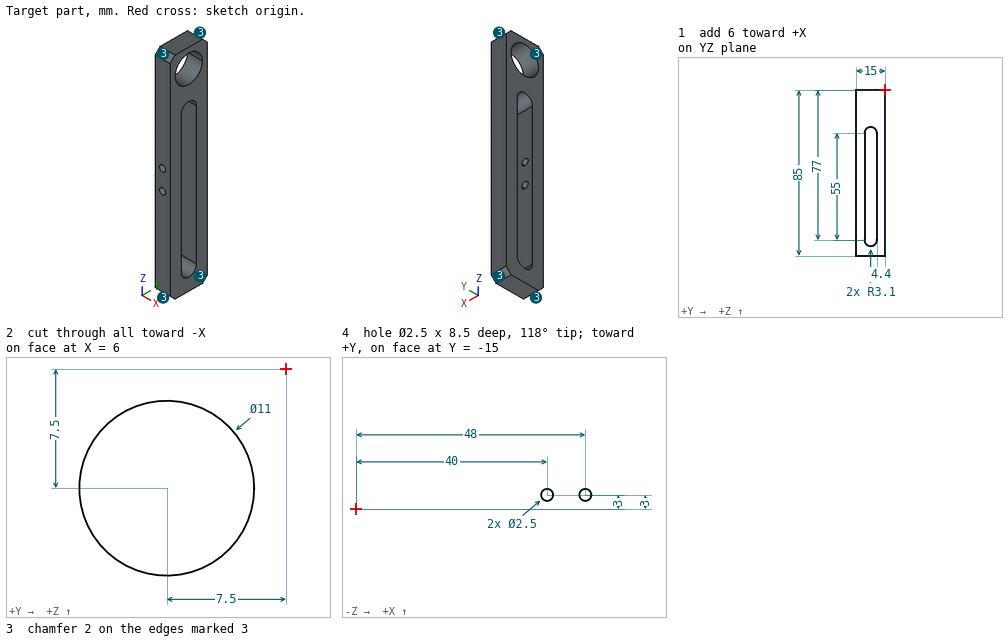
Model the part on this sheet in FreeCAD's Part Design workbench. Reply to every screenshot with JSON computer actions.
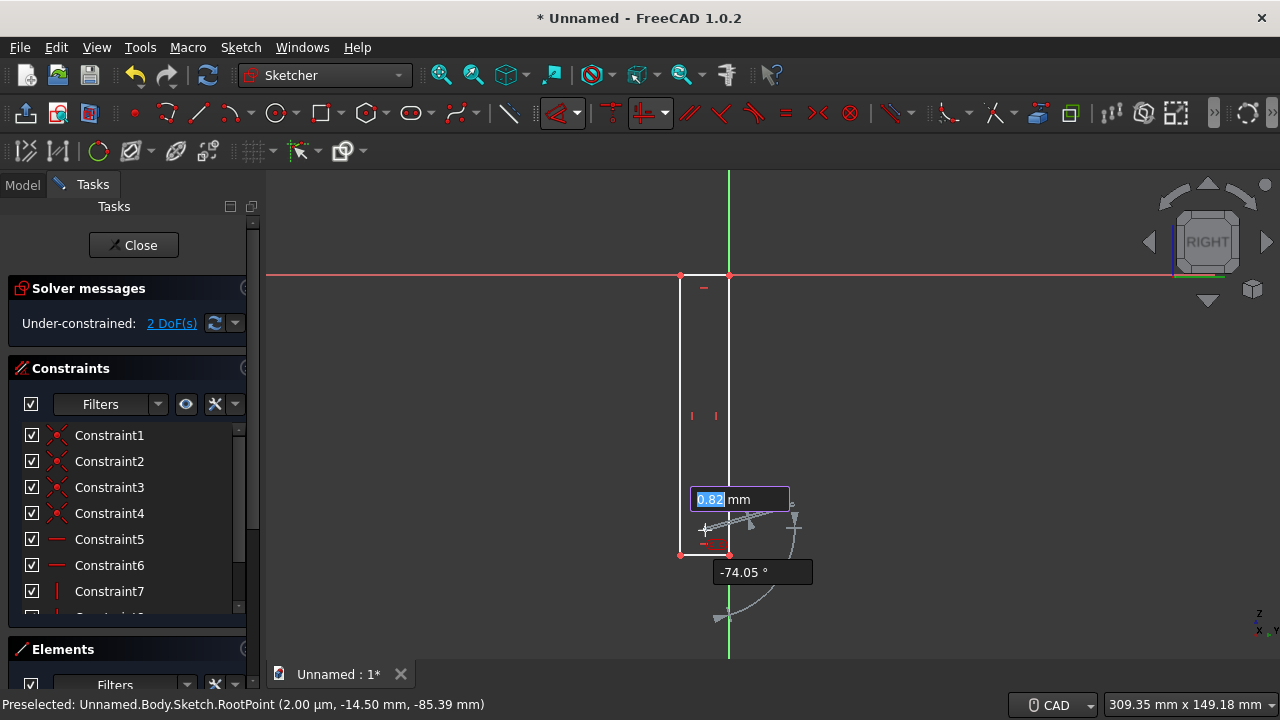
{"action": "left_click", "coordinate": [705, 348]}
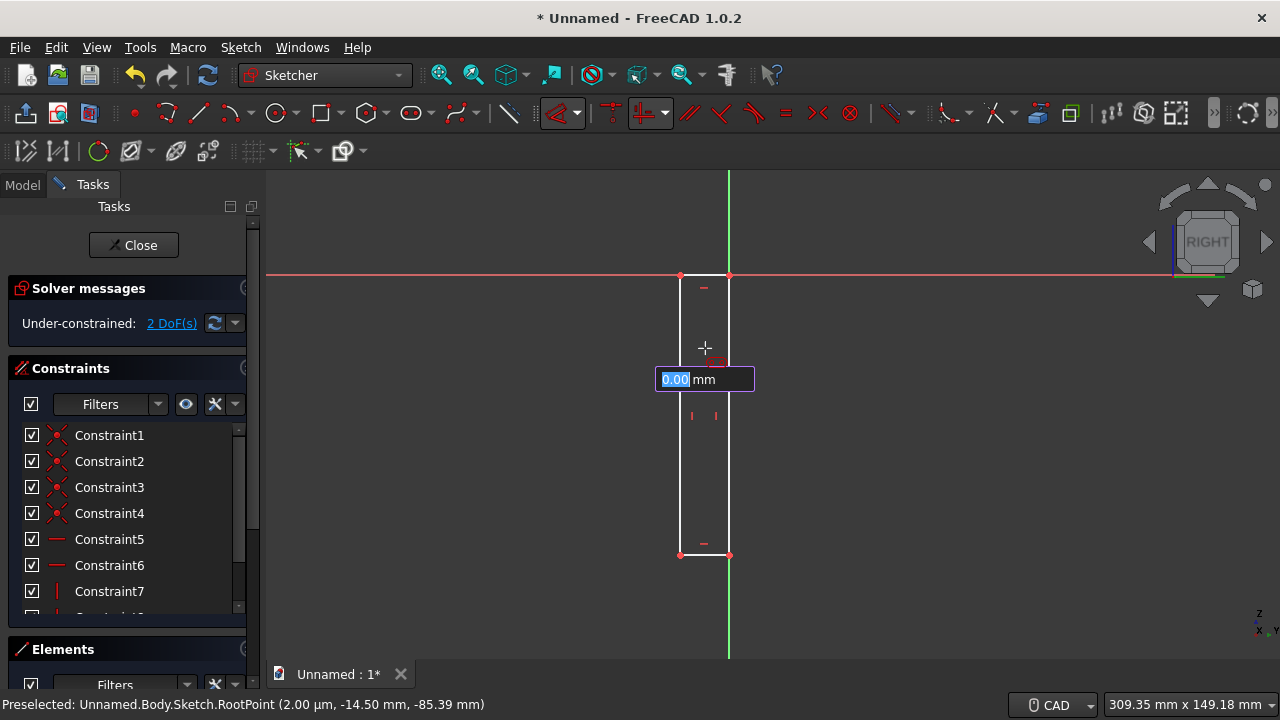
{"action": "scroll", "coordinate": [715, 438], "scroll_direction": "up", "scroll_amount": 3}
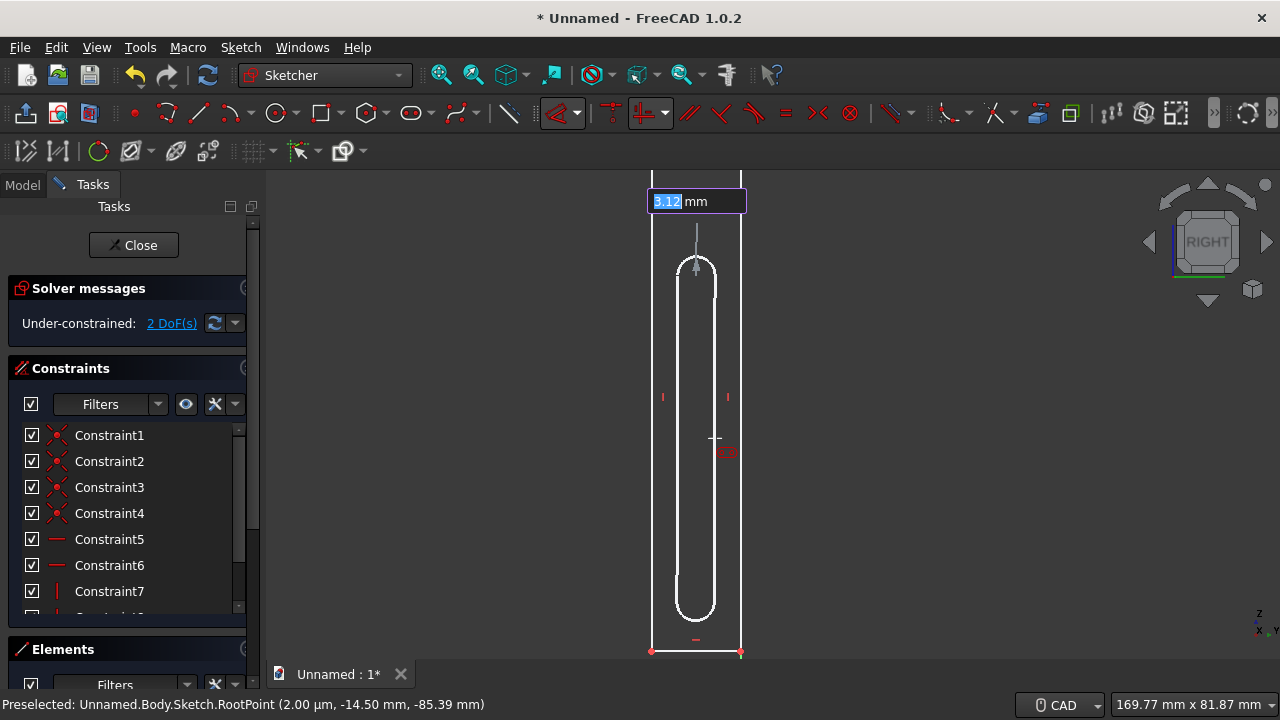
{"action": "left_click", "coordinate": [714, 437]}
{"action": "key", "text": "Escape"}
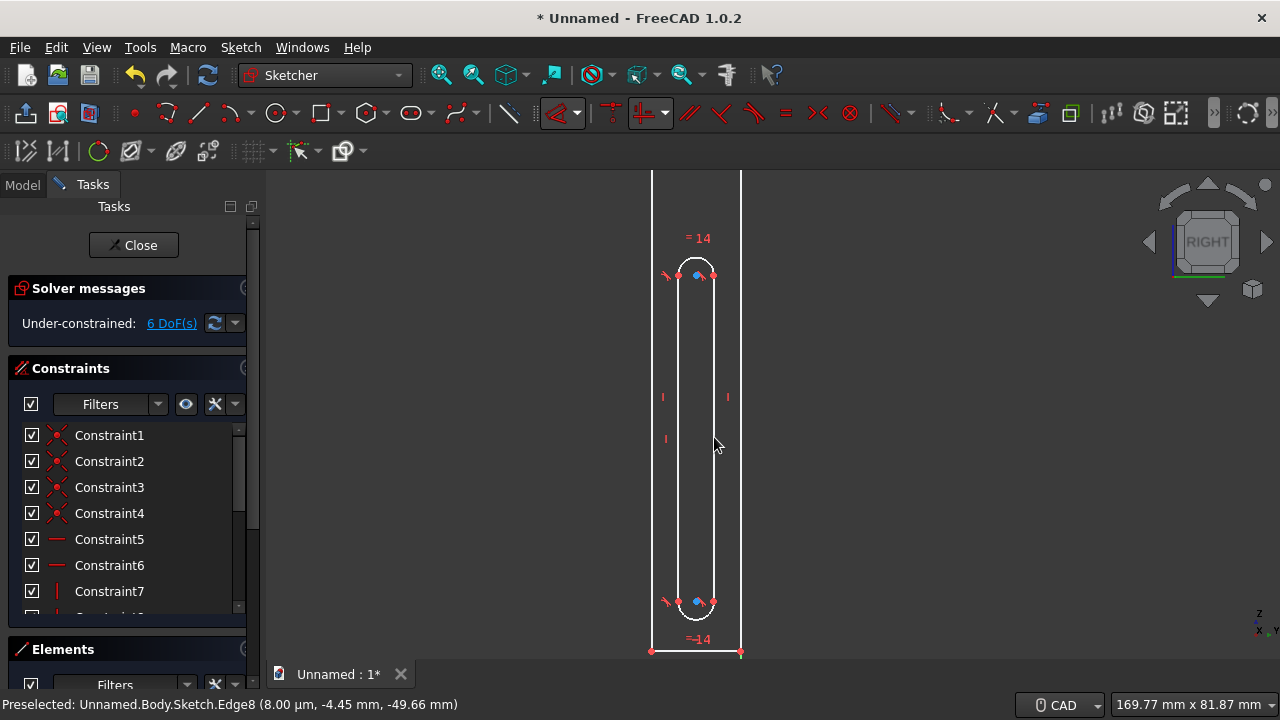
{"action": "key", "text": "d"}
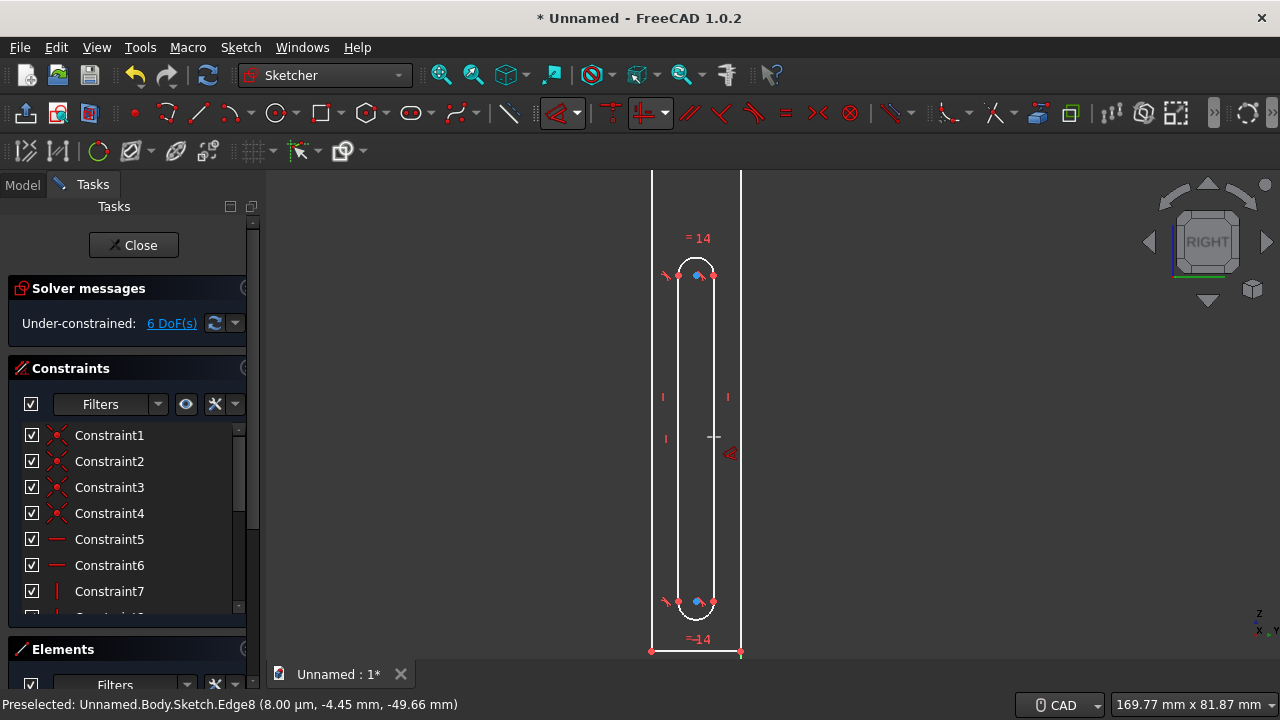
{"action": "scroll", "coordinate": [686, 616], "scroll_direction": "up", "scroll_amount": 4}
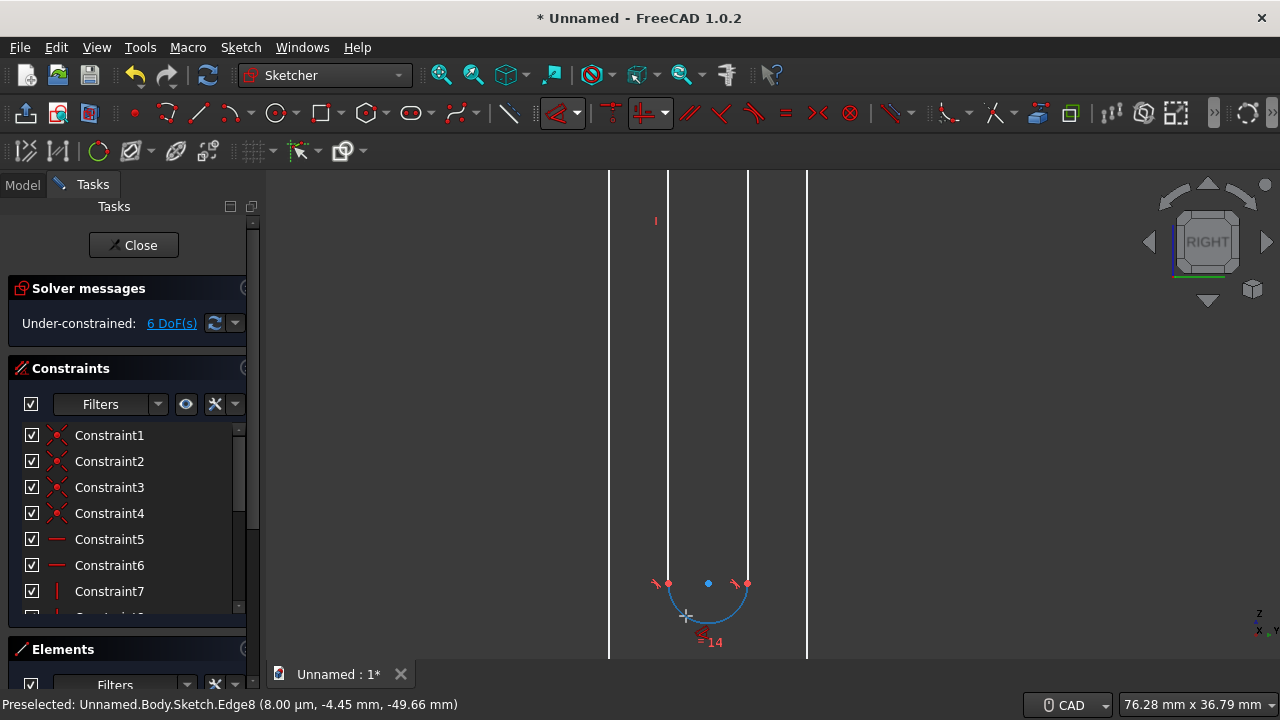
{"action": "left_click", "coordinate": [685, 616]}
{"action": "left_click", "coordinate": [644, 615]}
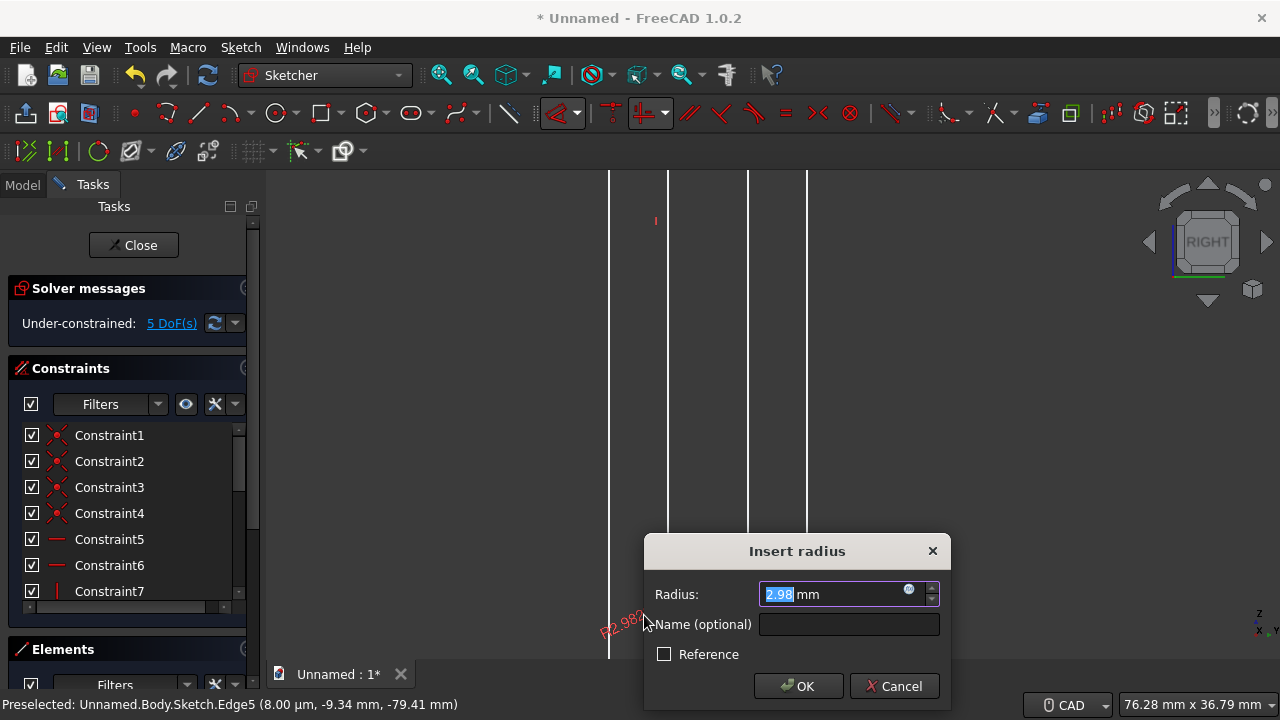
{"action": "type", "text": "3.1"}
{"action": "key", "text": "Return"}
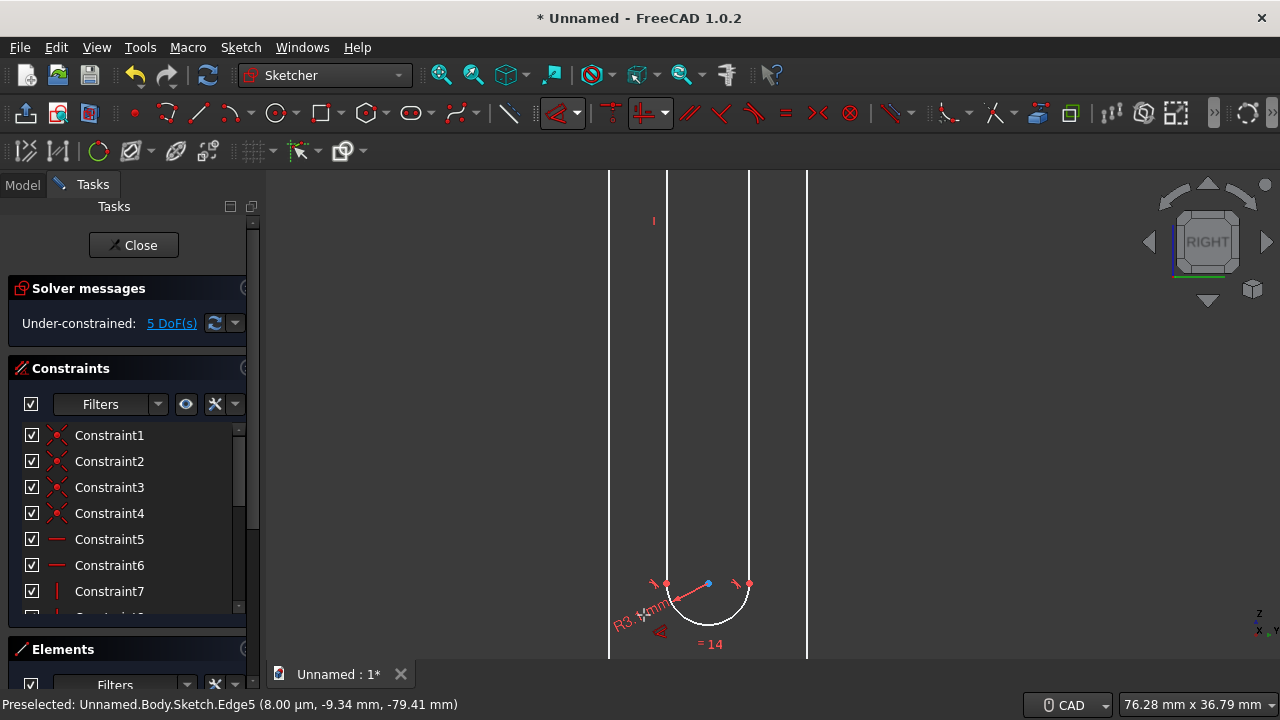
{"action": "scroll", "coordinate": [704, 510], "scroll_direction": "down", "scroll_amount": 7}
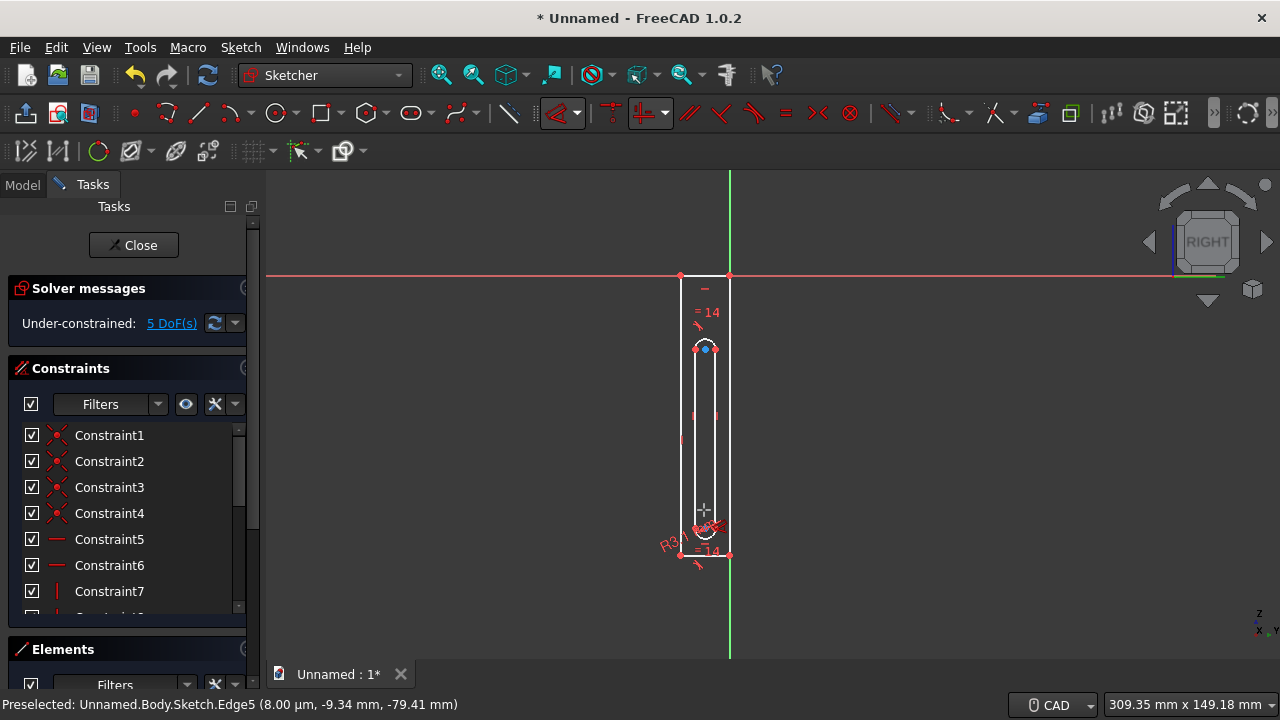
{"action": "left_click", "coordinate": [715, 276]}
{"action": "left_click", "coordinate": [705, 242]}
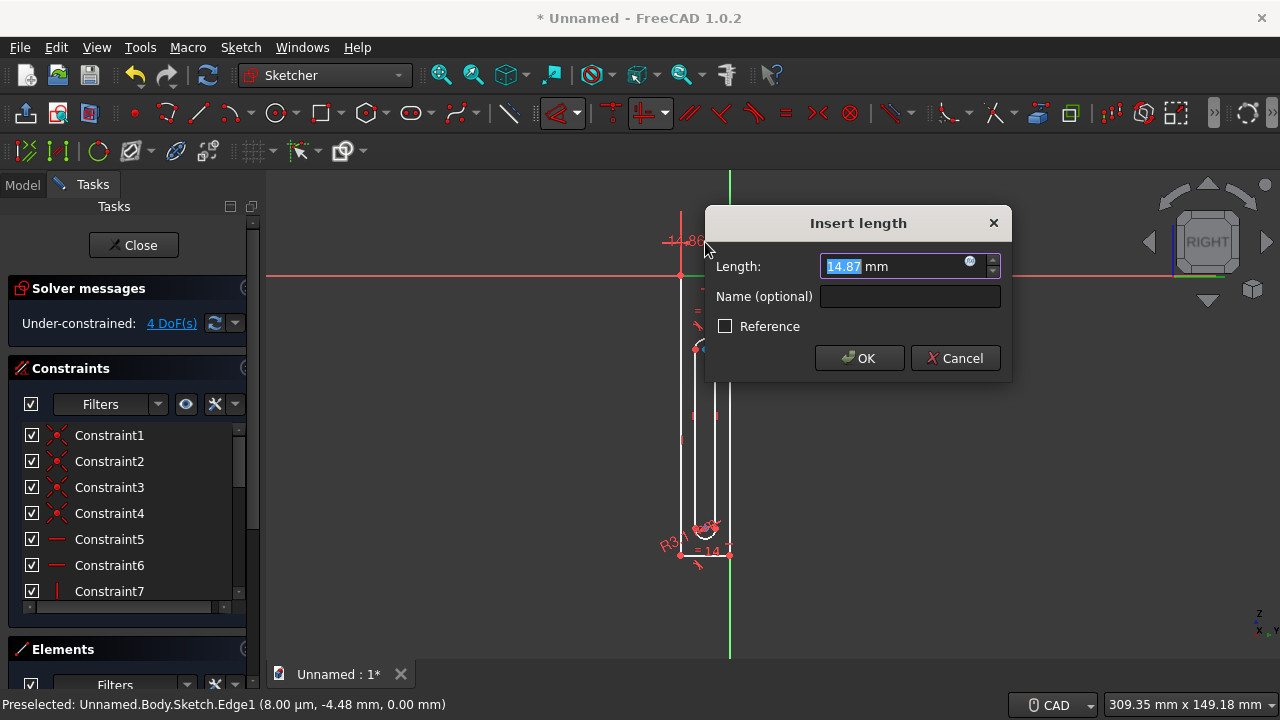
{"action": "type", "text": "15"}
{"action": "key", "text": "Return"}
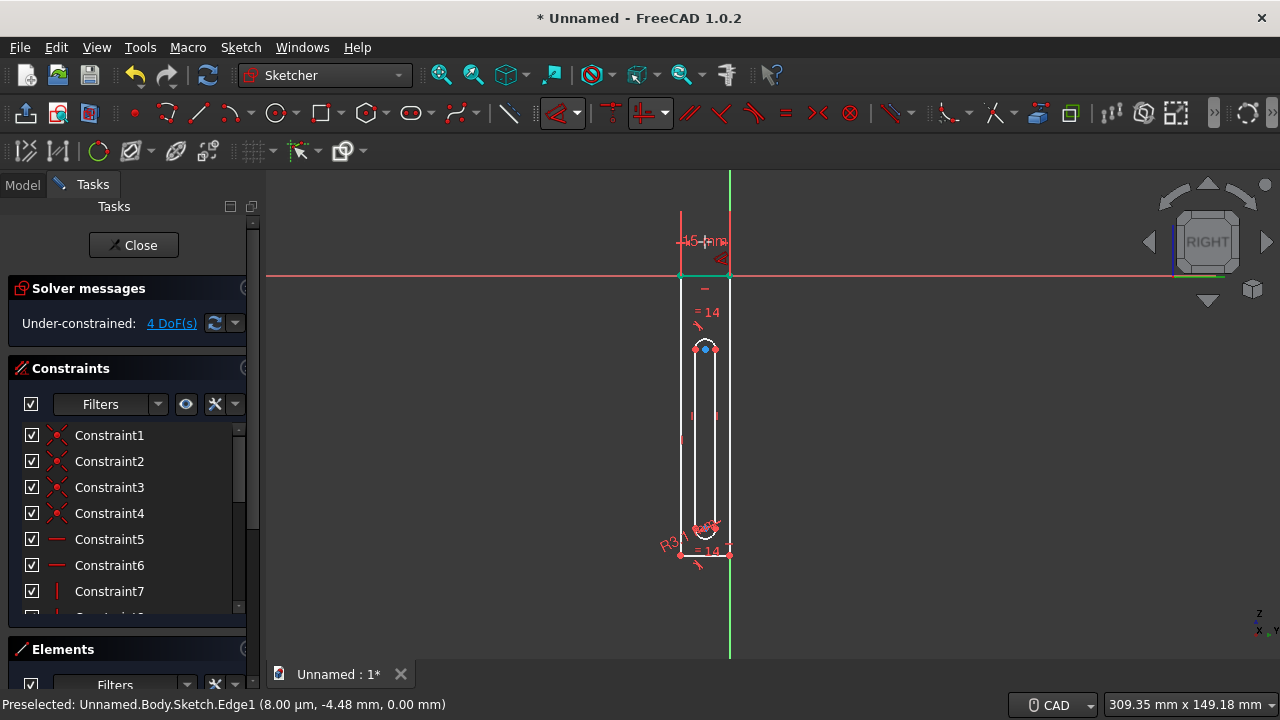
{"action": "left_click", "coordinate": [681, 360]}
{"action": "left_click", "coordinate": [647, 416]}